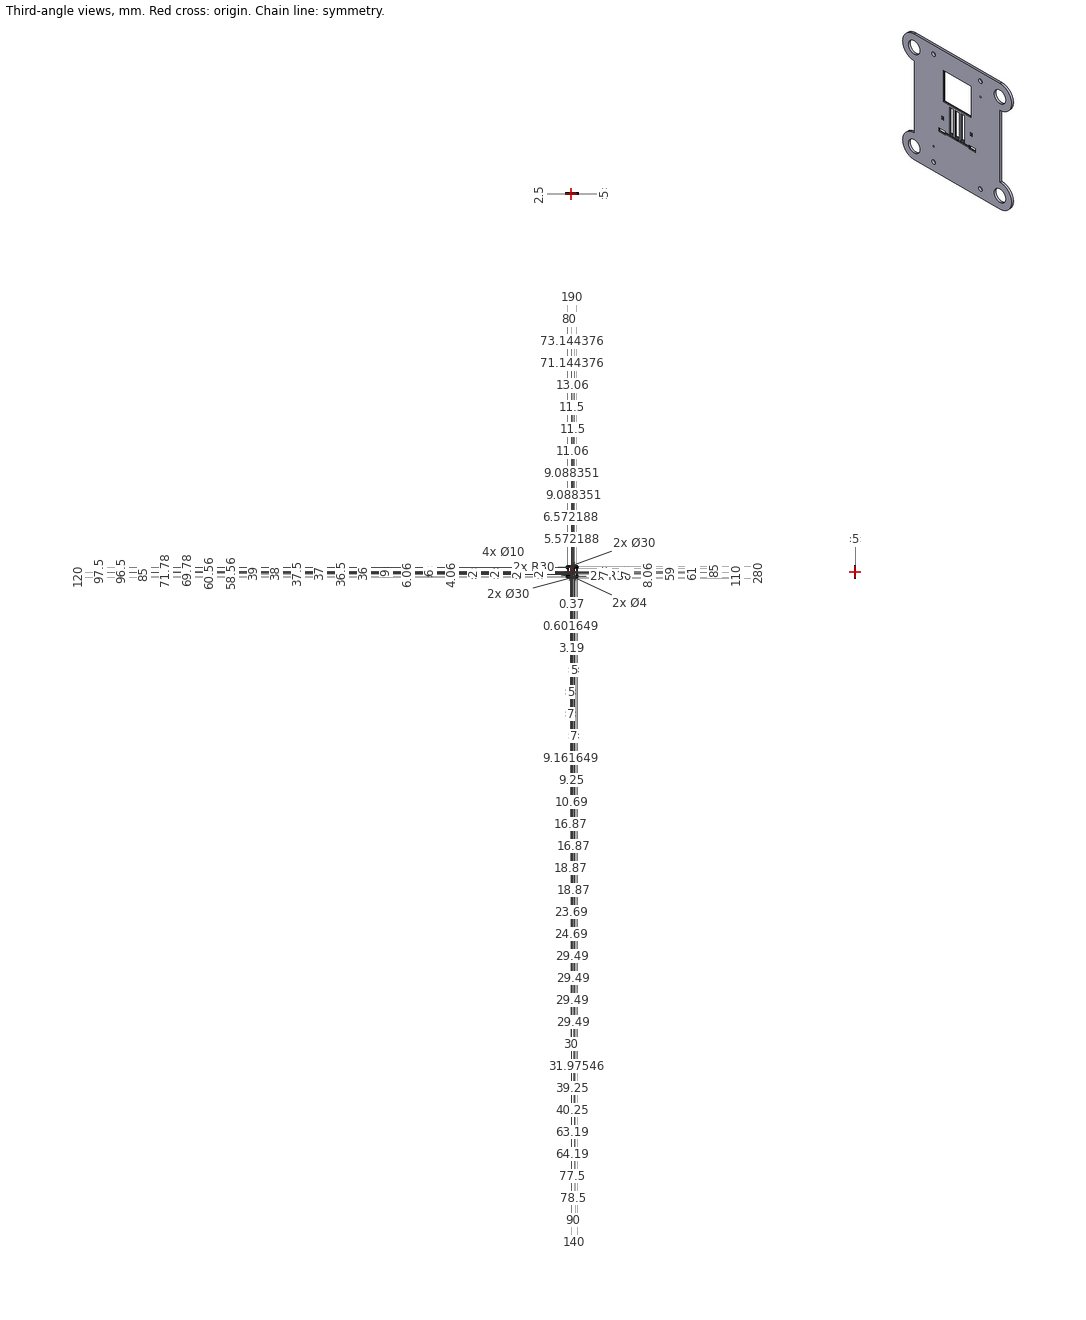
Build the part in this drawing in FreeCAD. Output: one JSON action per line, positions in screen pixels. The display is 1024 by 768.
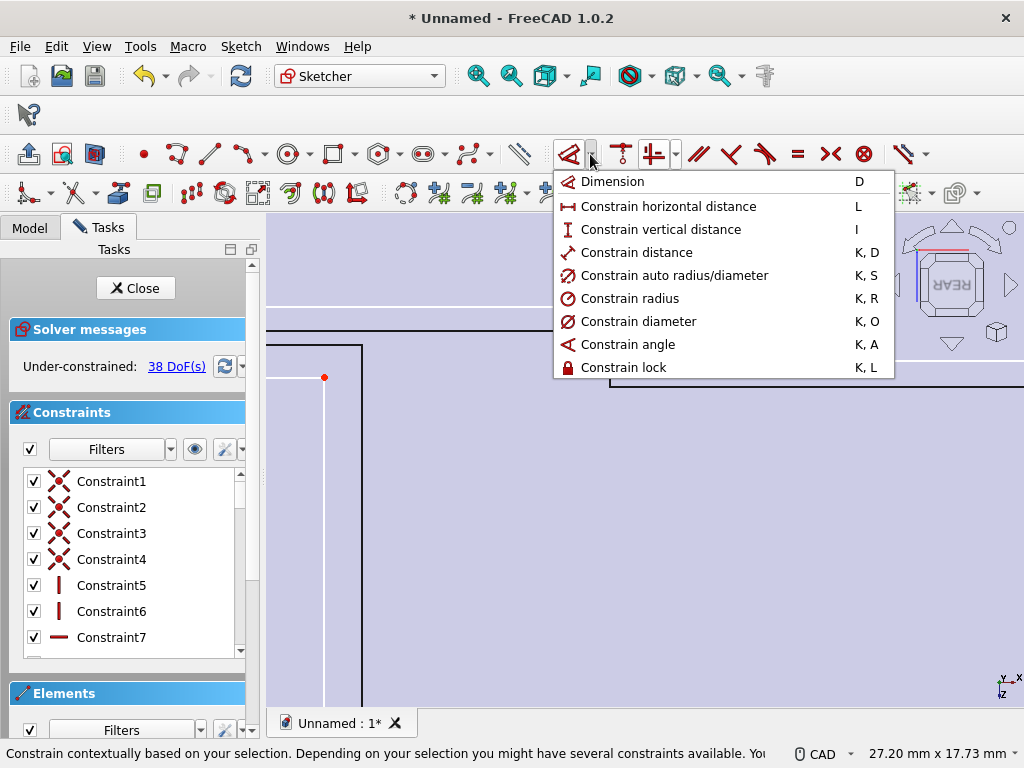
{"action": "left_click", "coordinate": [724, 230]}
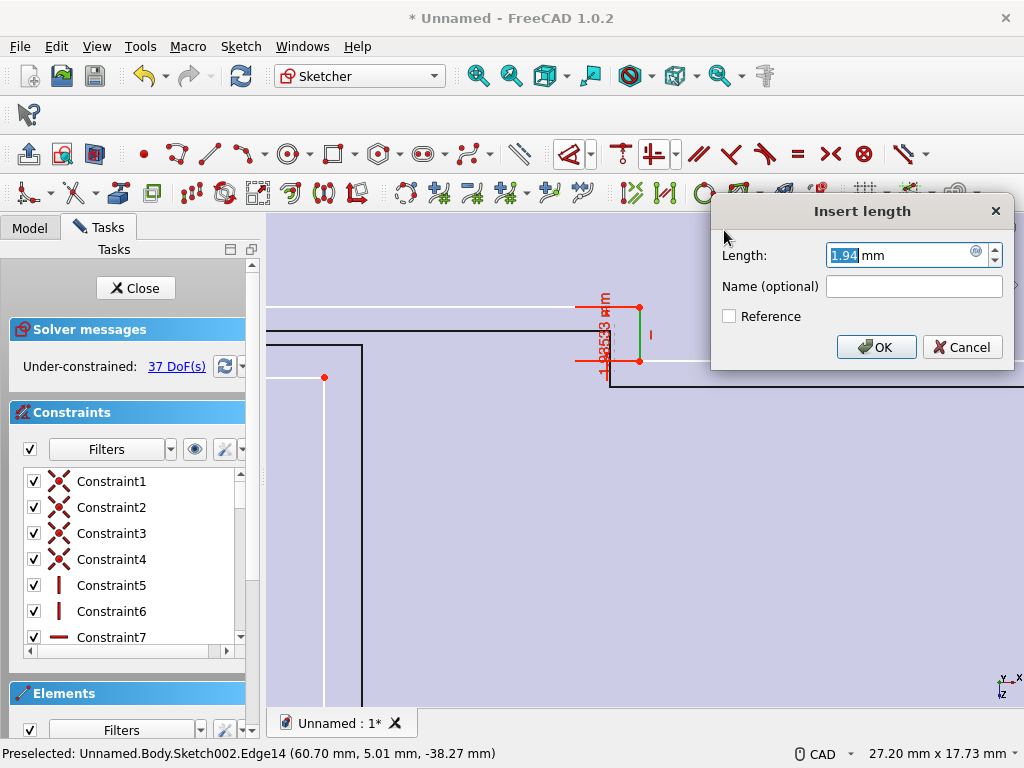
{"action": "type", "text": "2"}
{"action": "key", "text": "Return"}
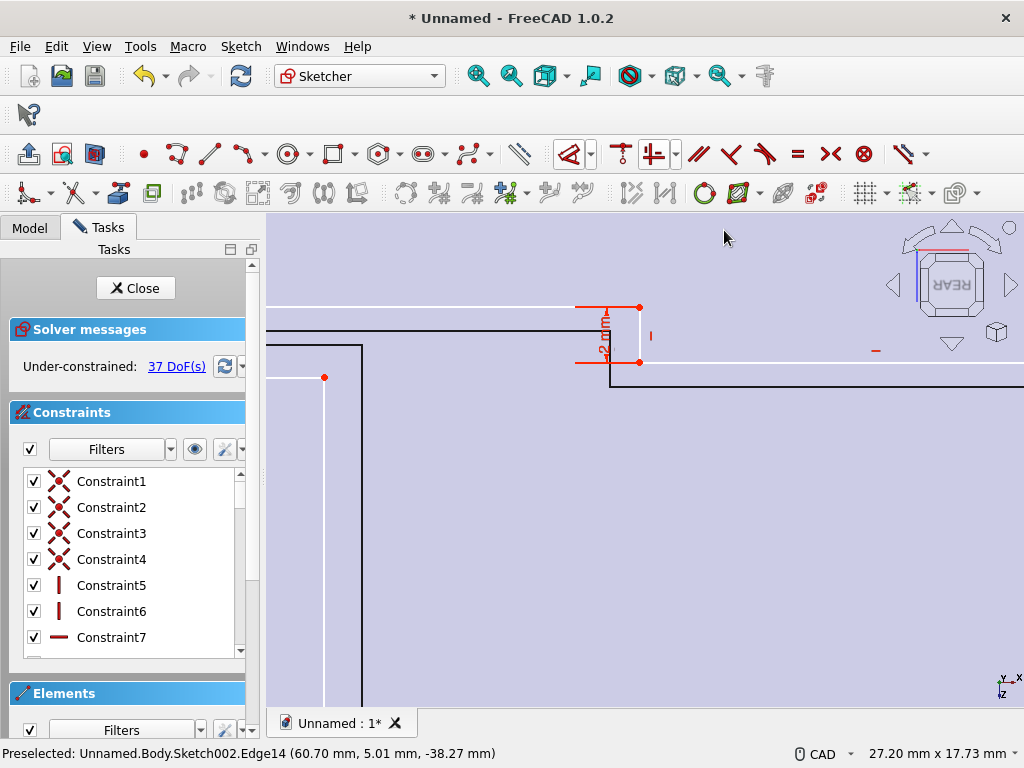
{"action": "scroll", "coordinate": [640, 328], "scroll_direction": "down", "scroll_amount": 13}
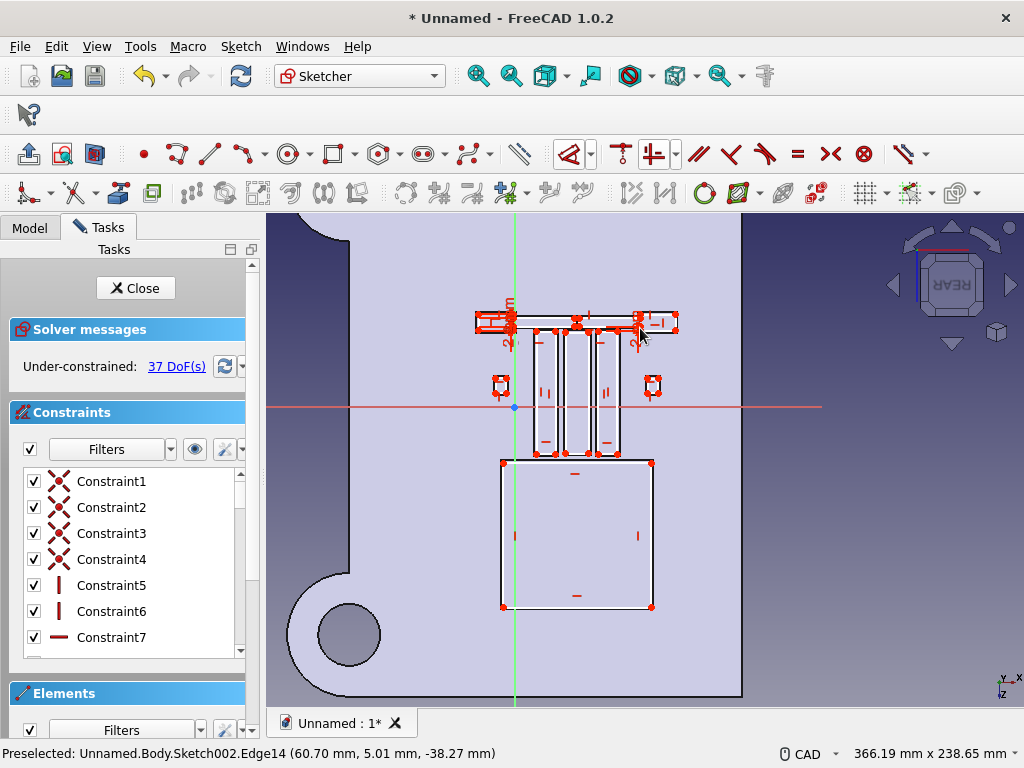
{"action": "scroll", "coordinate": [640, 316], "scroll_direction": "up", "scroll_amount": 13}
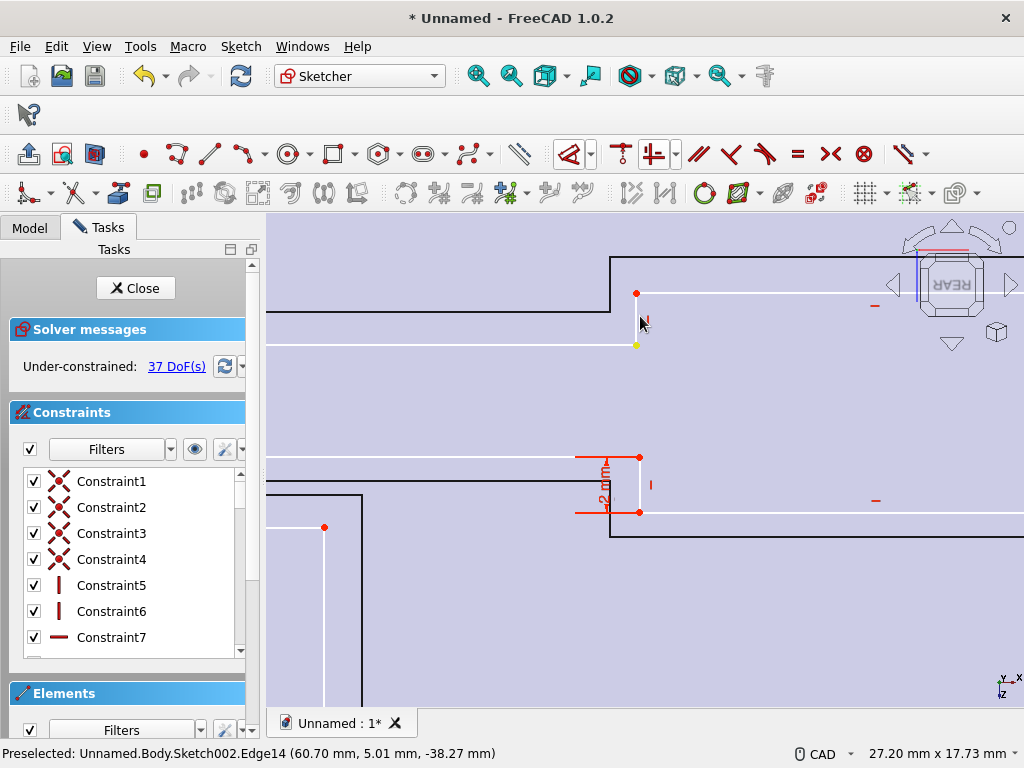
{"action": "left_click", "coordinate": [636, 309]}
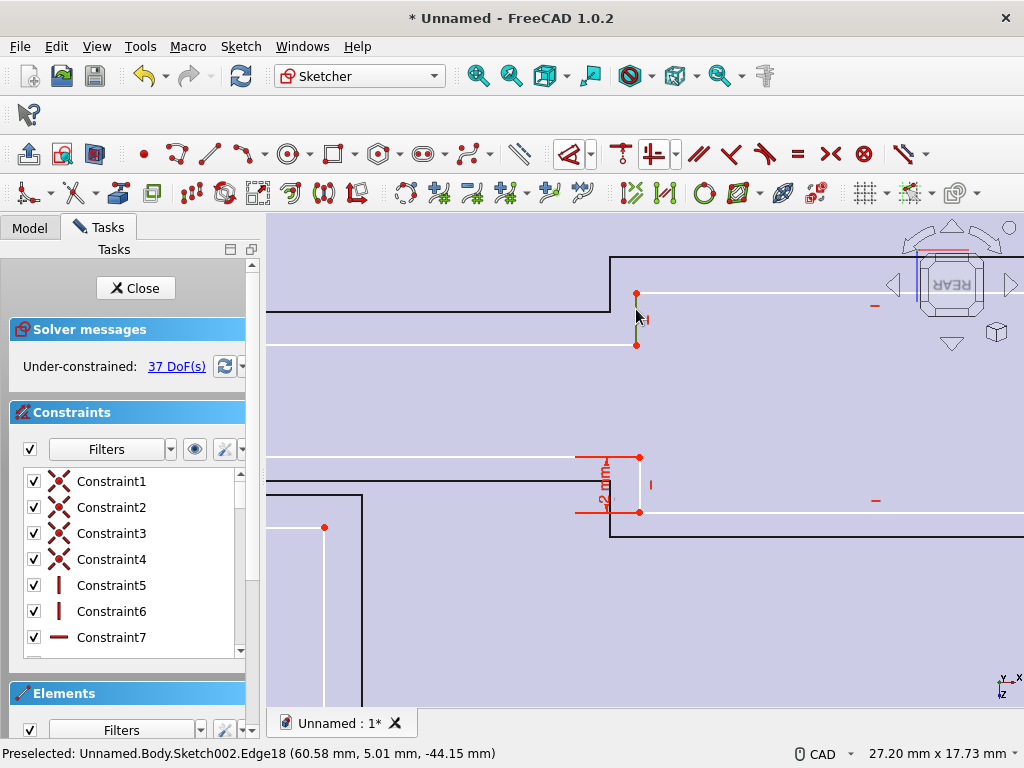
{"action": "key", "text": "i"}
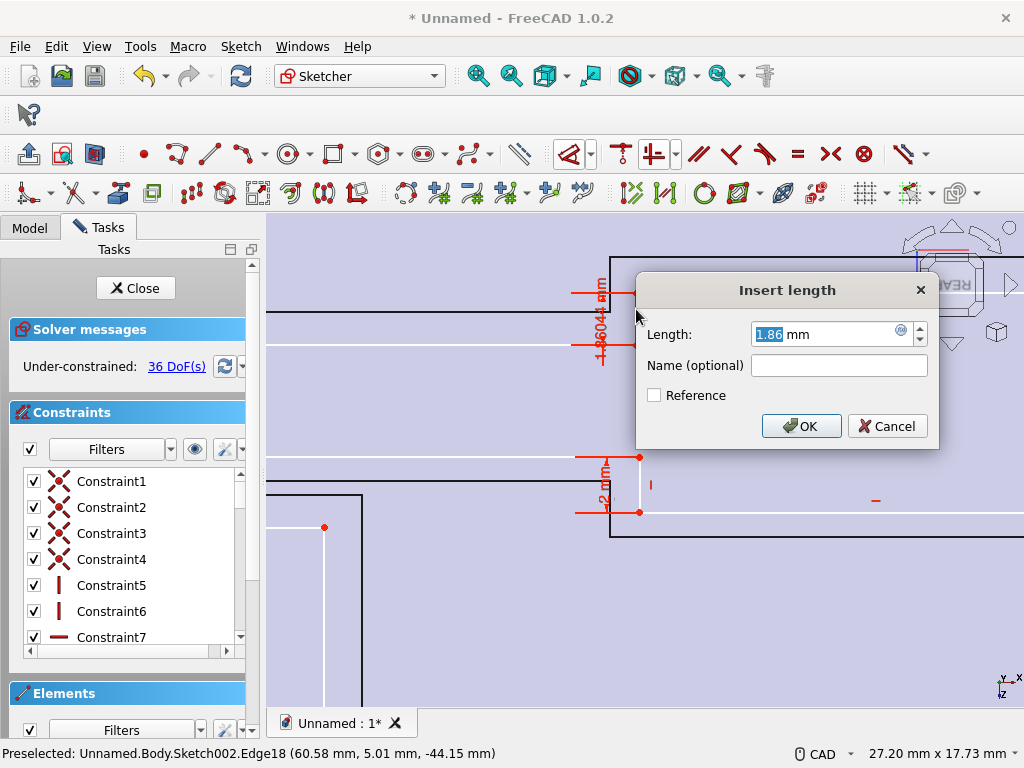
{"action": "type", "text": "2"}
{"action": "key", "text": "Return"}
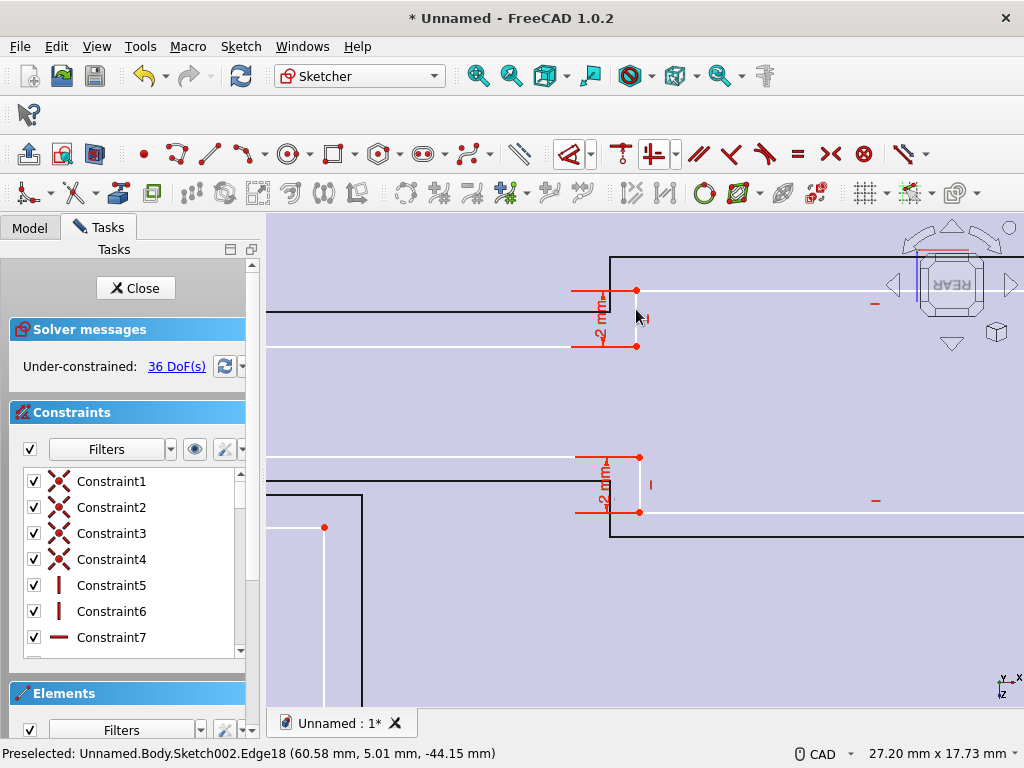
{"action": "scroll", "coordinate": [640, 316], "scroll_direction": "down", "scroll_amount": 13}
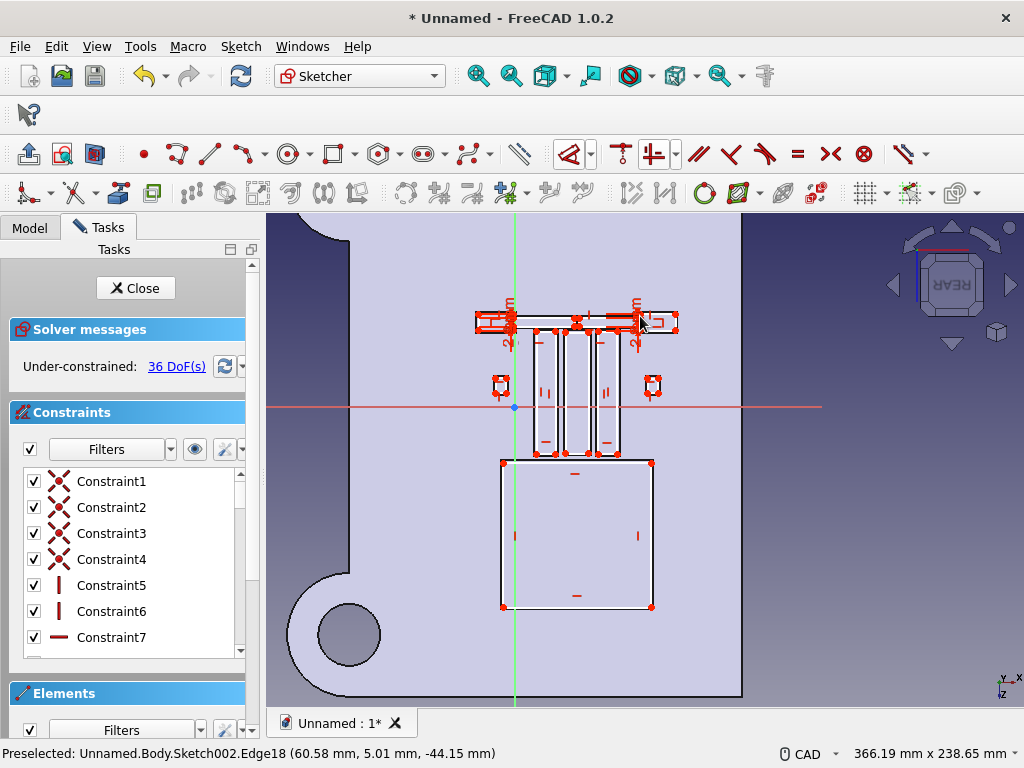
{"action": "scroll", "coordinate": [648, 383], "scroll_direction": "up", "scroll_amount": 6}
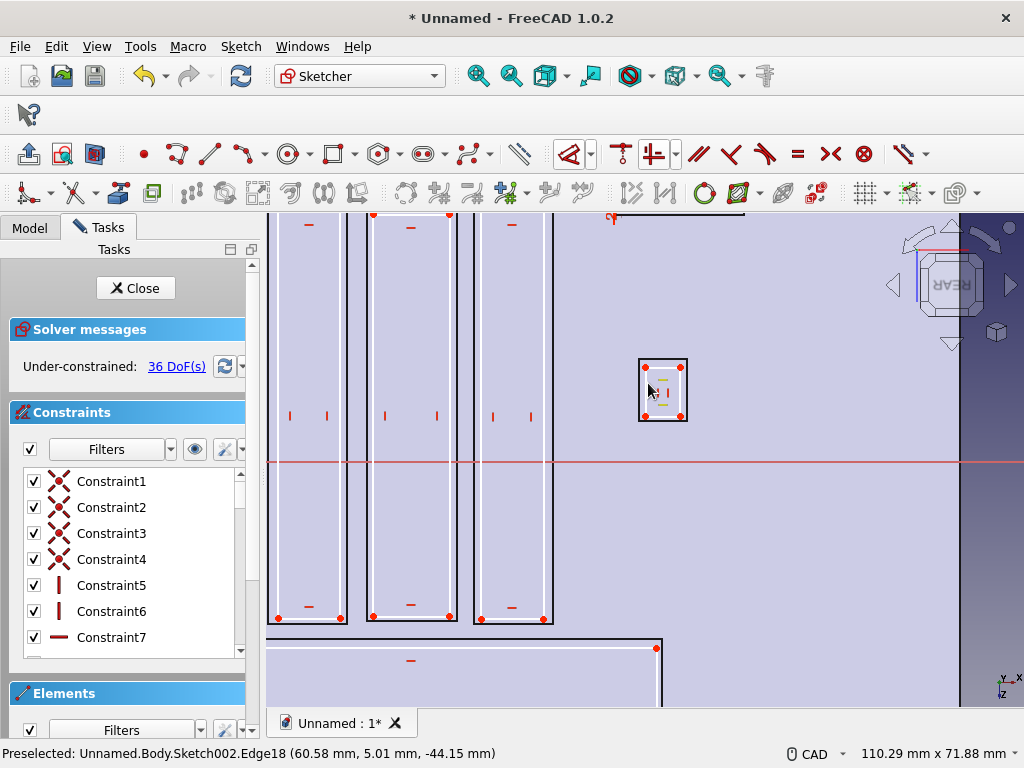
{"action": "left_click", "coordinate": [646, 382]}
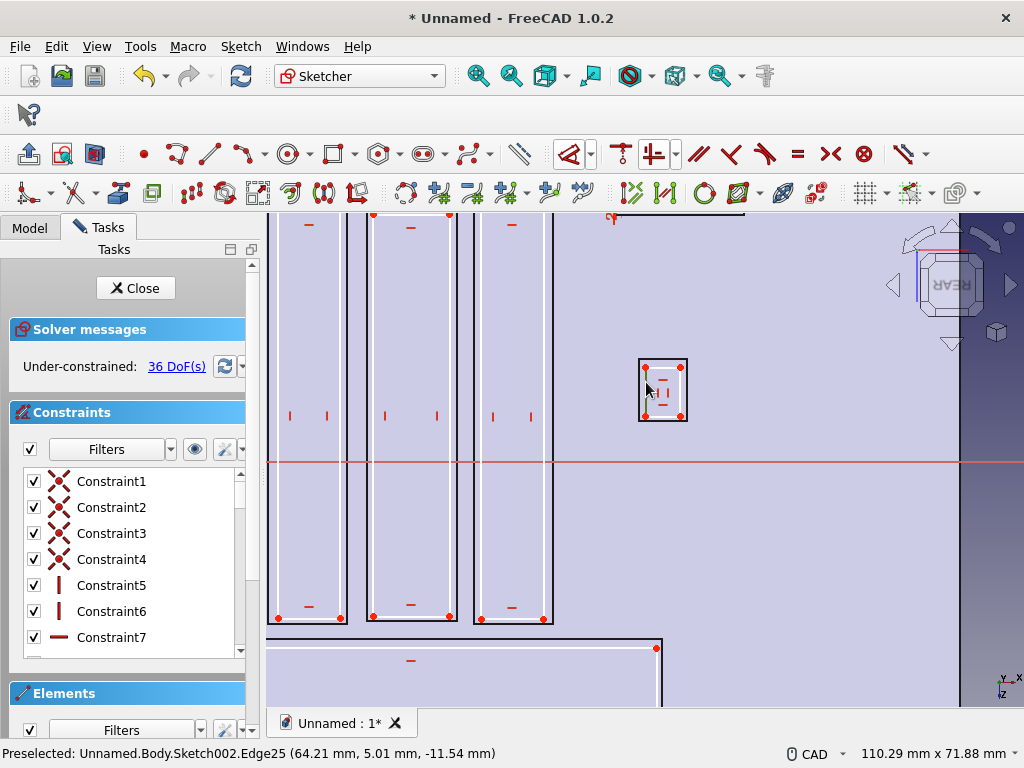
{"action": "left_click", "coordinate": [590, 154]}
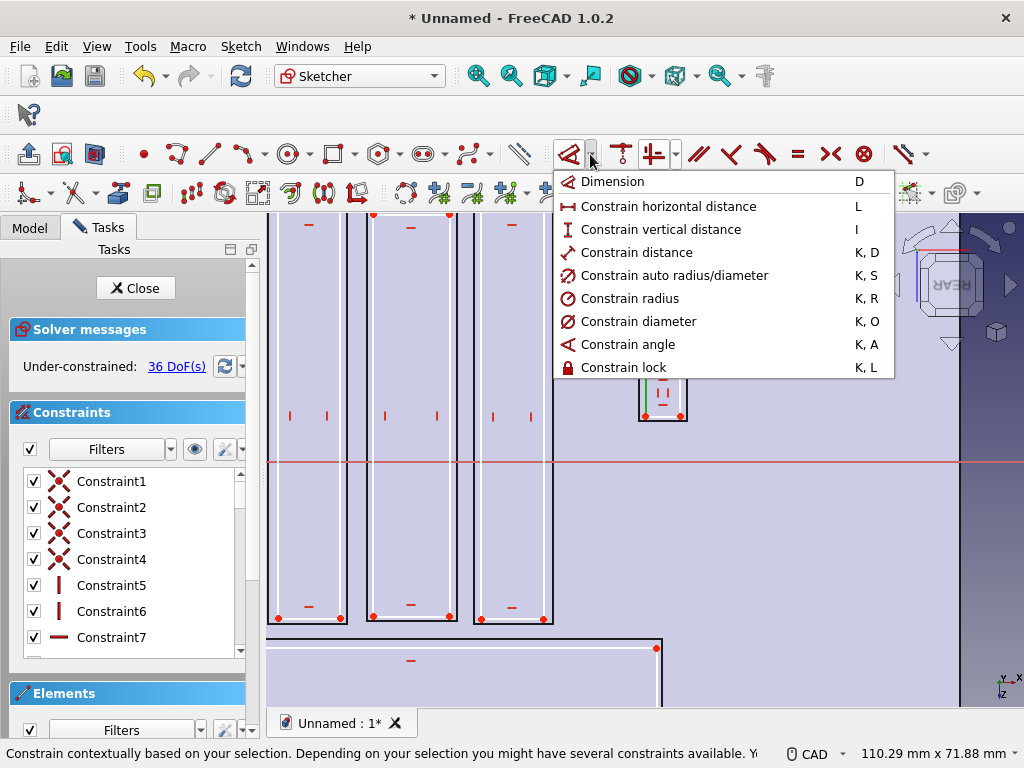
{"action": "left_click", "coordinate": [724, 230]}